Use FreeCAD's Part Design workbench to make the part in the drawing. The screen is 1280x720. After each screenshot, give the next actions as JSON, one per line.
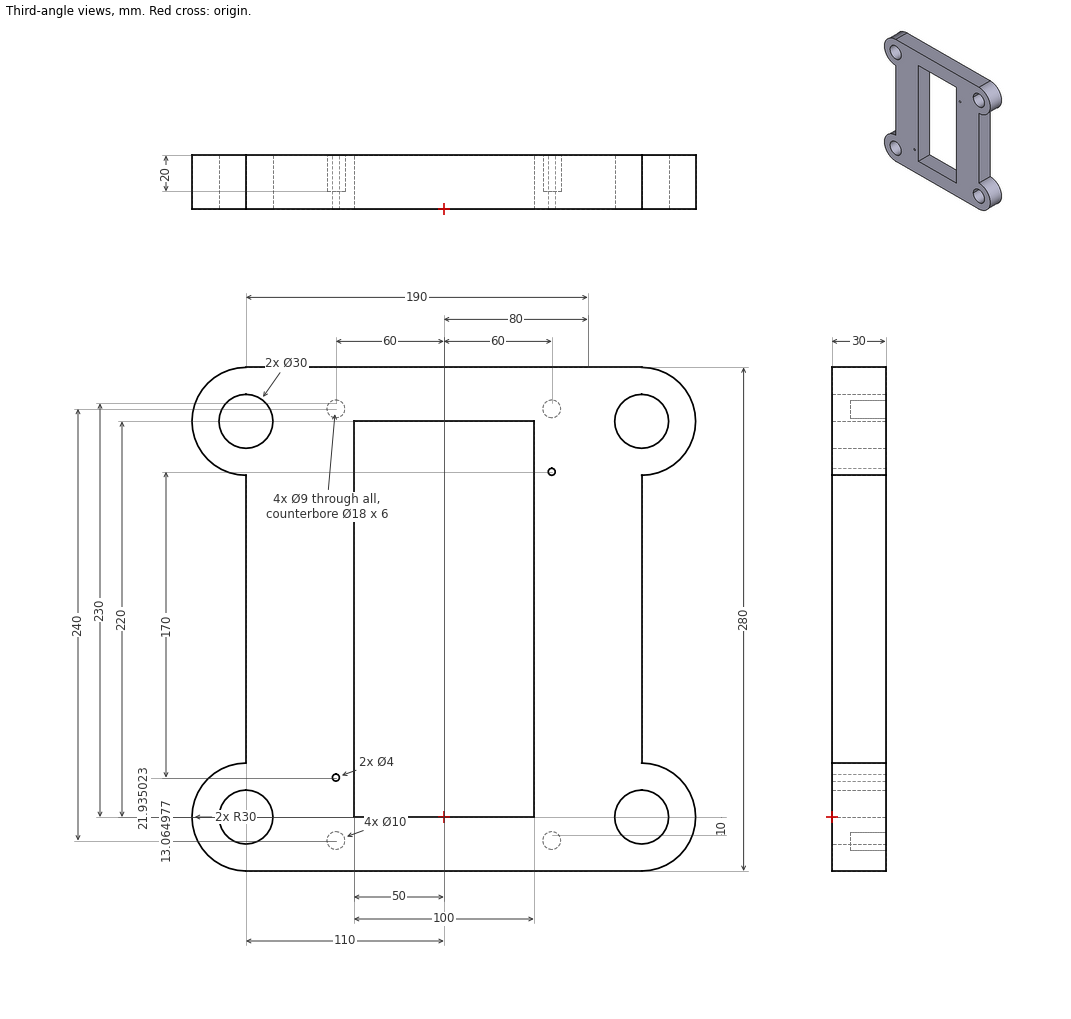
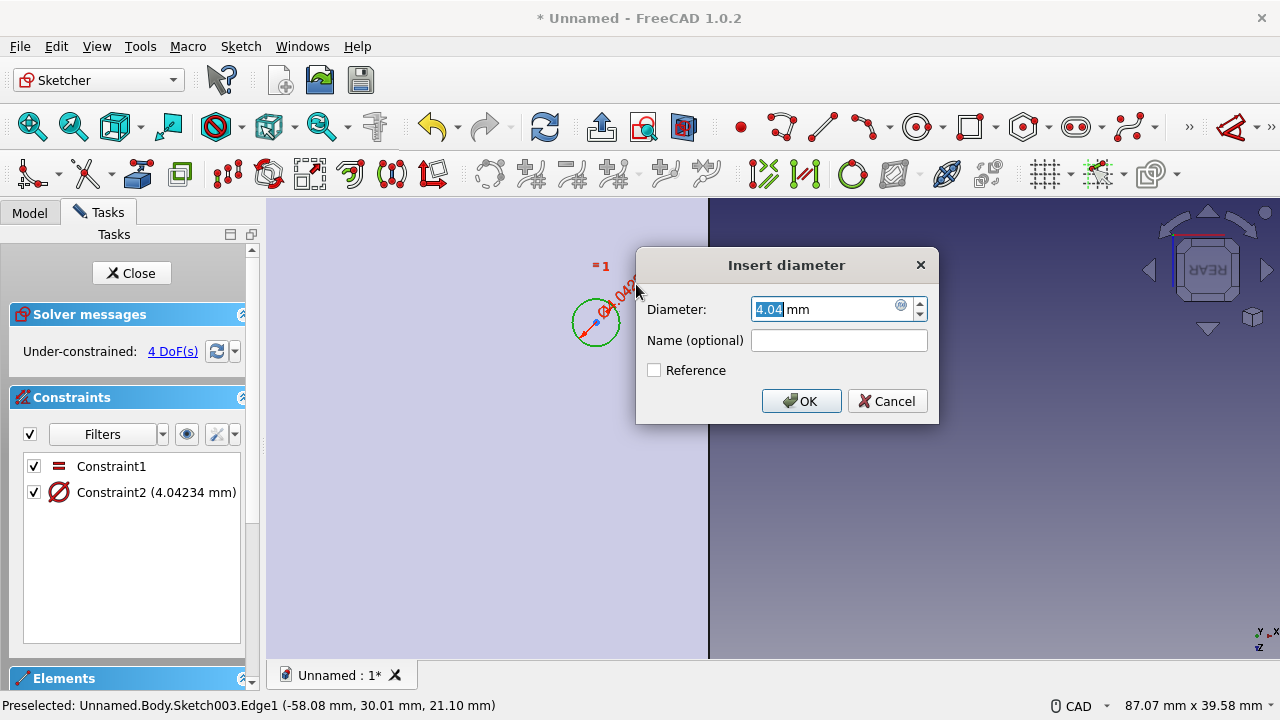
{"action": "type", "text": "4"}
{"action": "key", "text": "Return"}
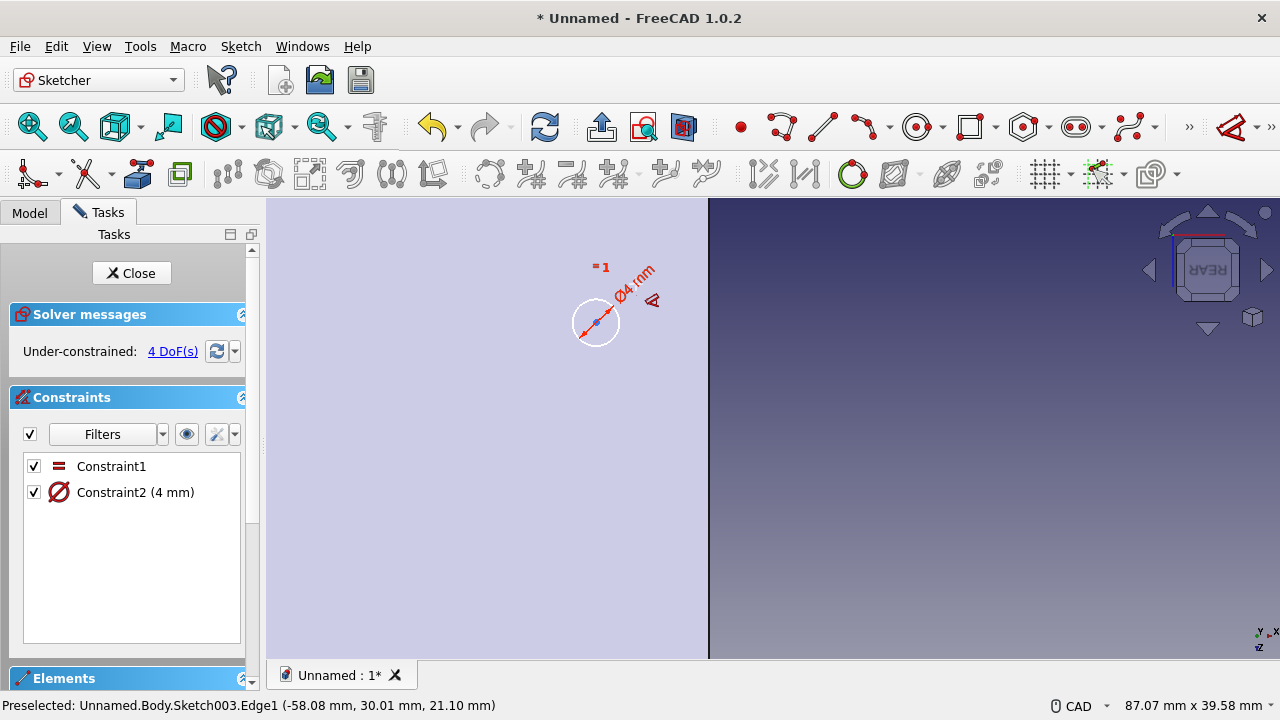
{"action": "scroll", "coordinate": [613, 309], "scroll_direction": "down", "scroll_amount": 10}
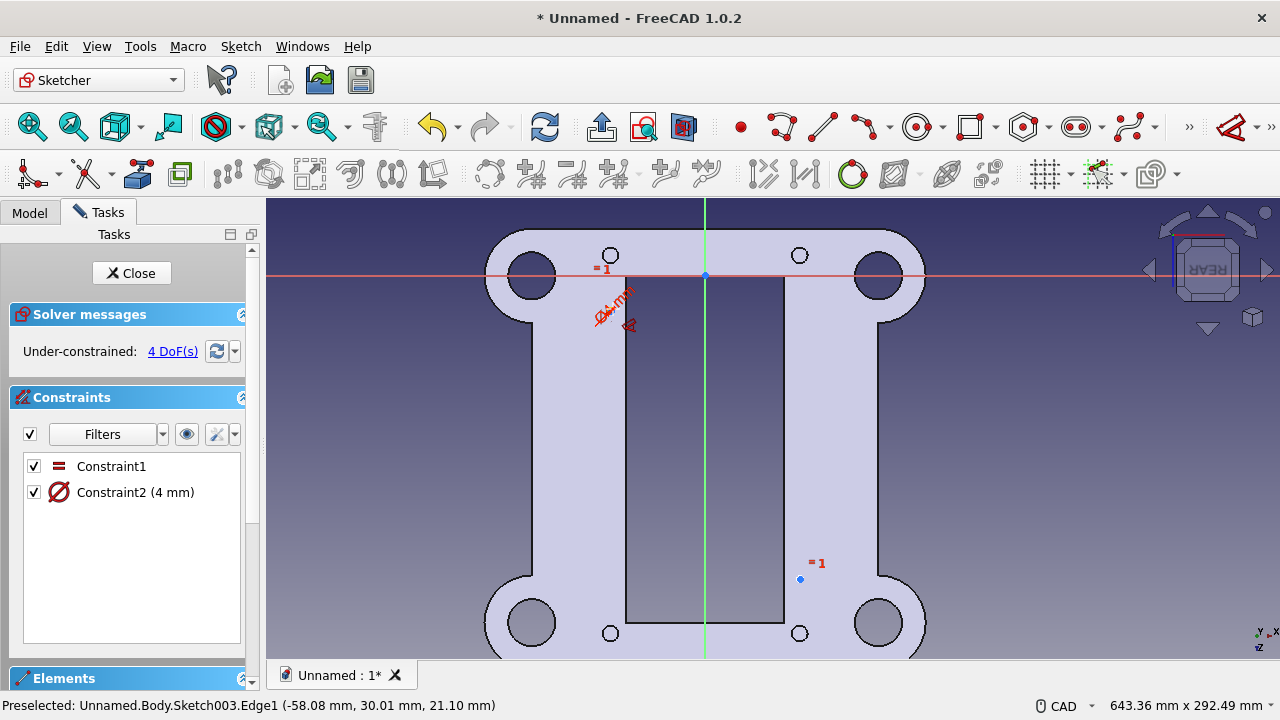
{"action": "left_click", "coordinate": [611, 311]}
{"action": "left_click", "coordinate": [658, 242]}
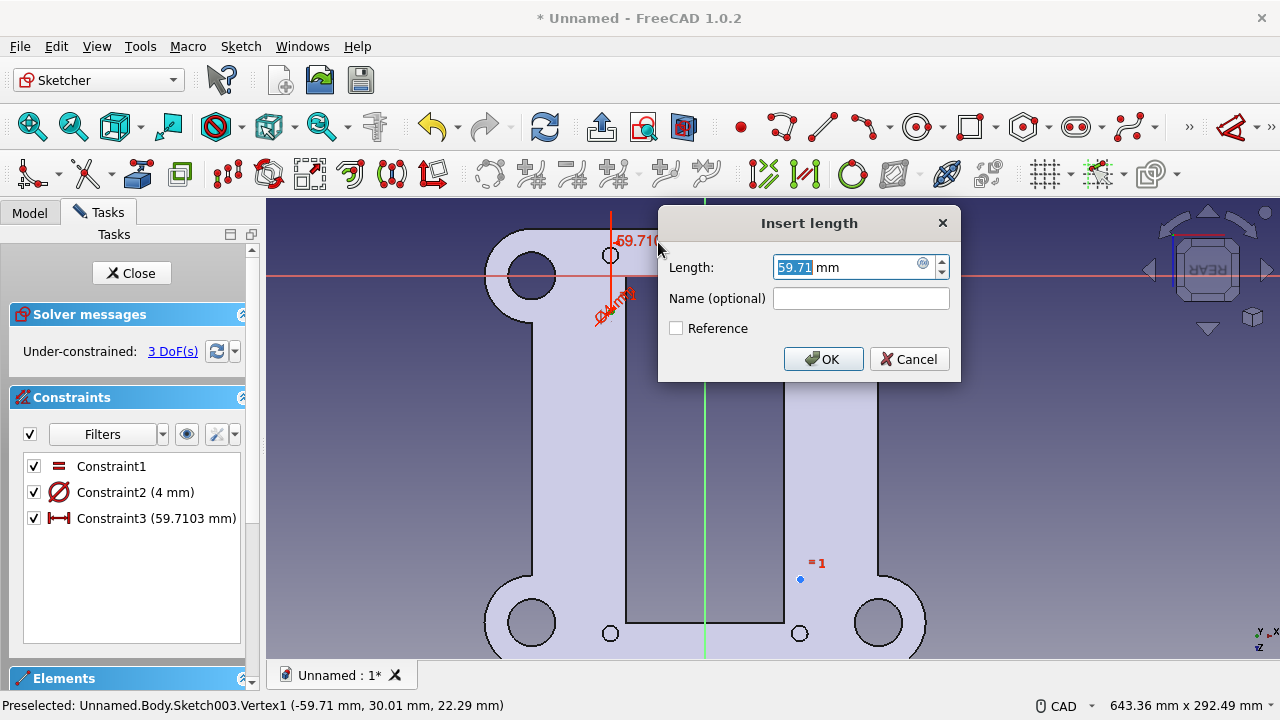
{"action": "type", "text": "60"}
{"action": "key", "text": "Return"}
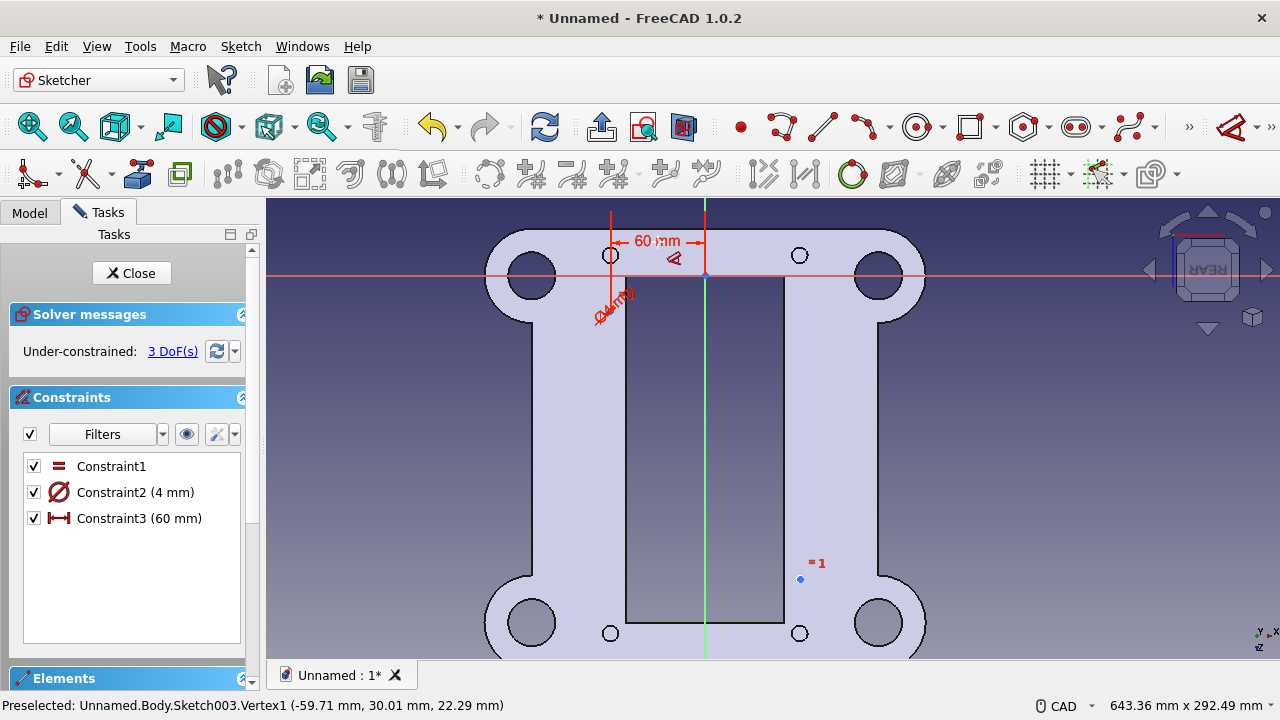
{"action": "left_click", "coordinate": [800, 579]}
{"action": "left_click", "coordinate": [753, 242]}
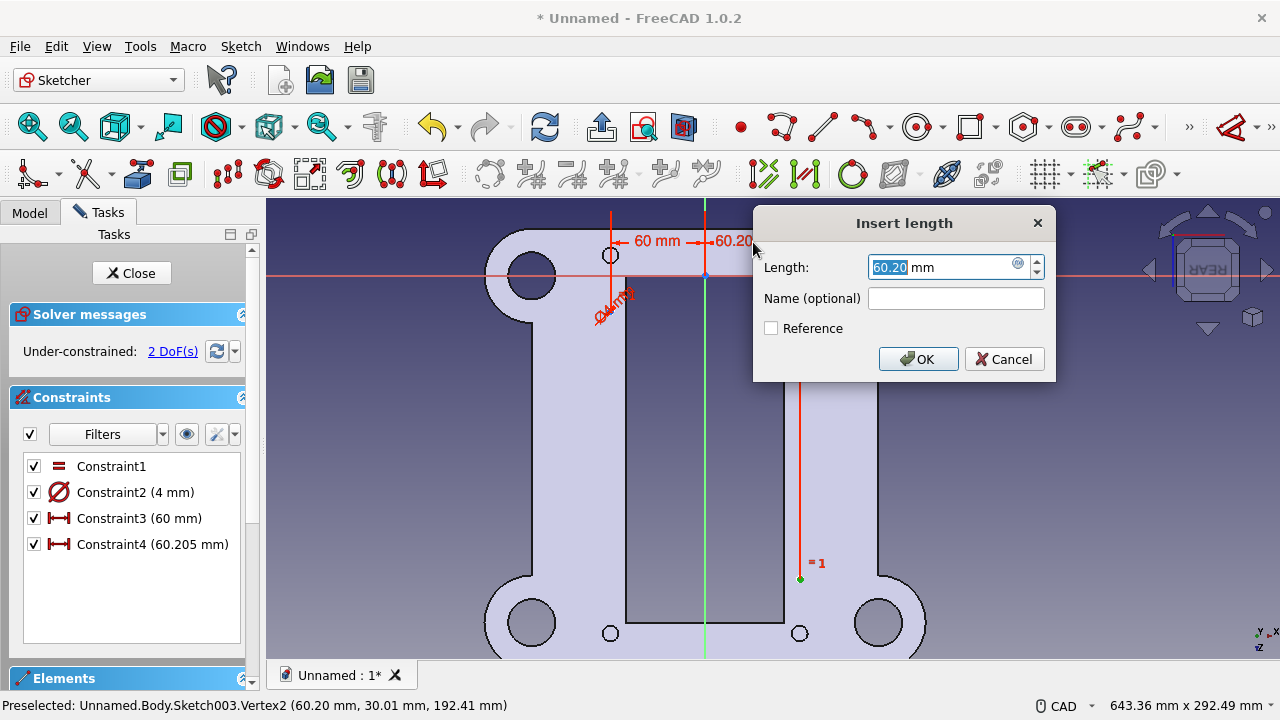
{"action": "type", "text": "60"}
{"action": "key", "text": "Return"}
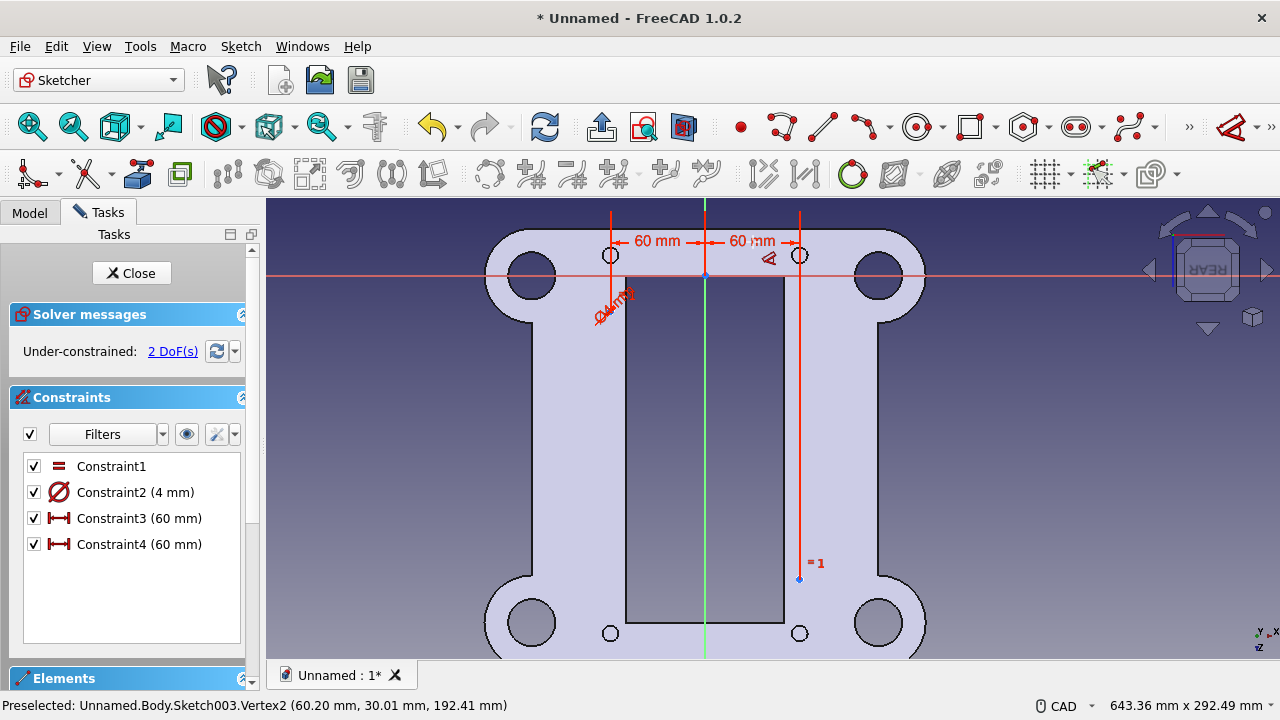
{"action": "left_click", "coordinate": [611, 311]}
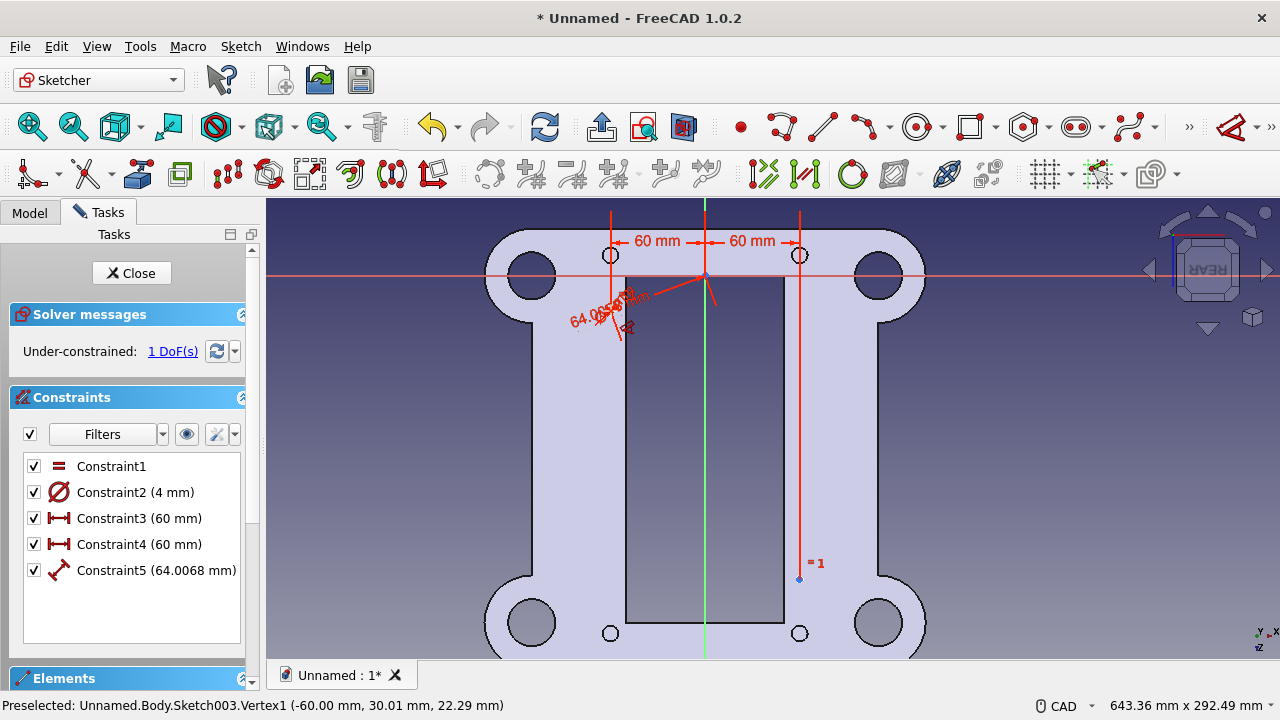
{"action": "left_click", "coordinate": [800, 579]}
{"action": "left_click", "coordinate": [834, 445]}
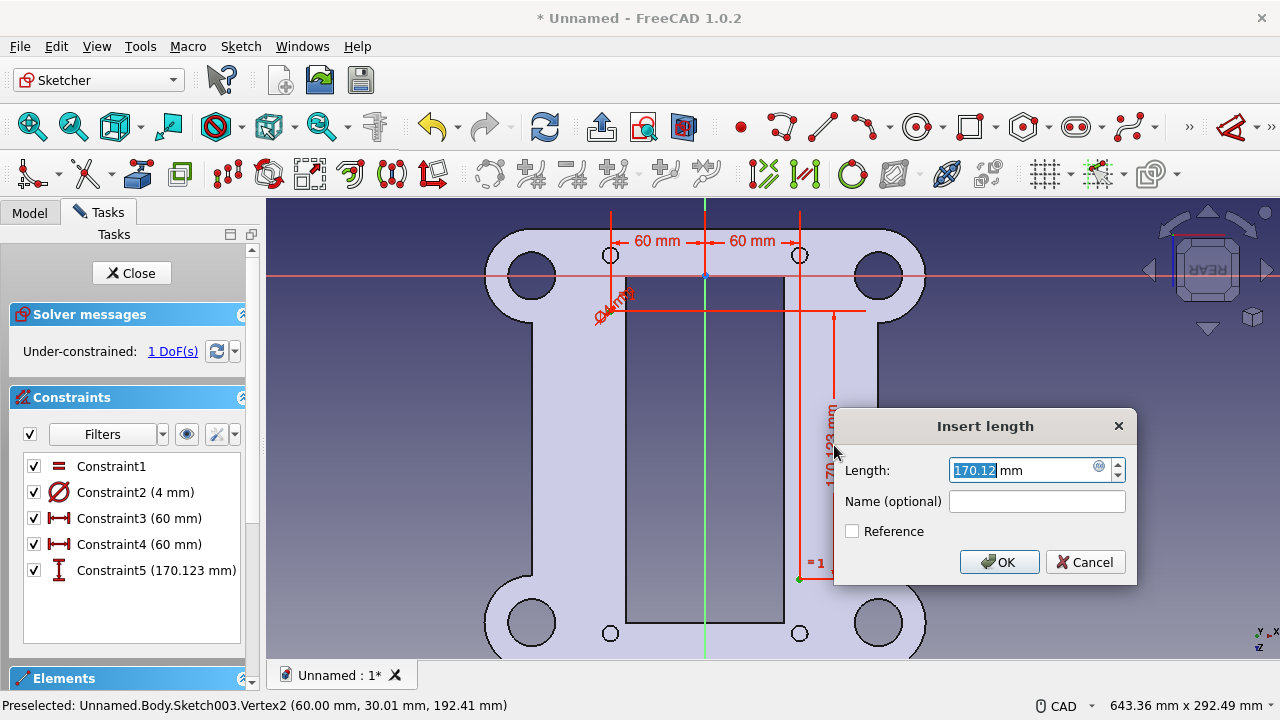
{"action": "type", "text": "170"}
{"action": "key", "text": "Return"}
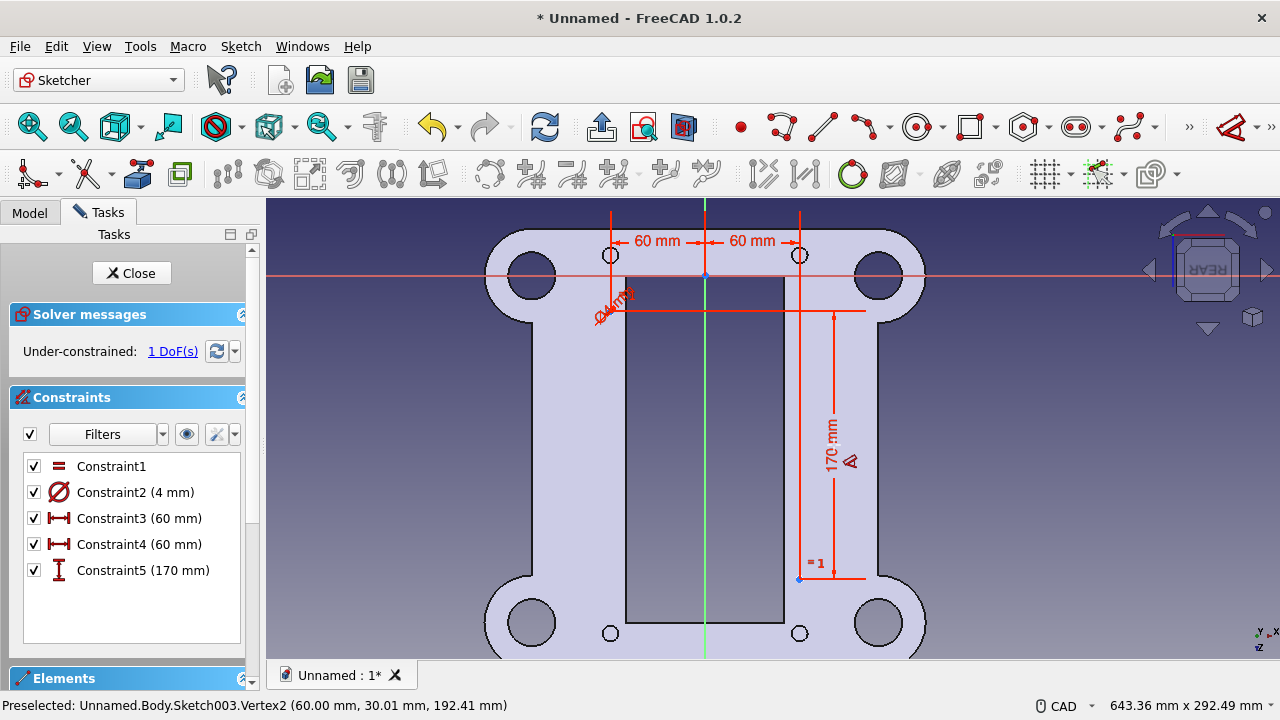
{"action": "left_click", "coordinate": [611, 311]}
{"action": "left_click", "coordinate": [739, 294]}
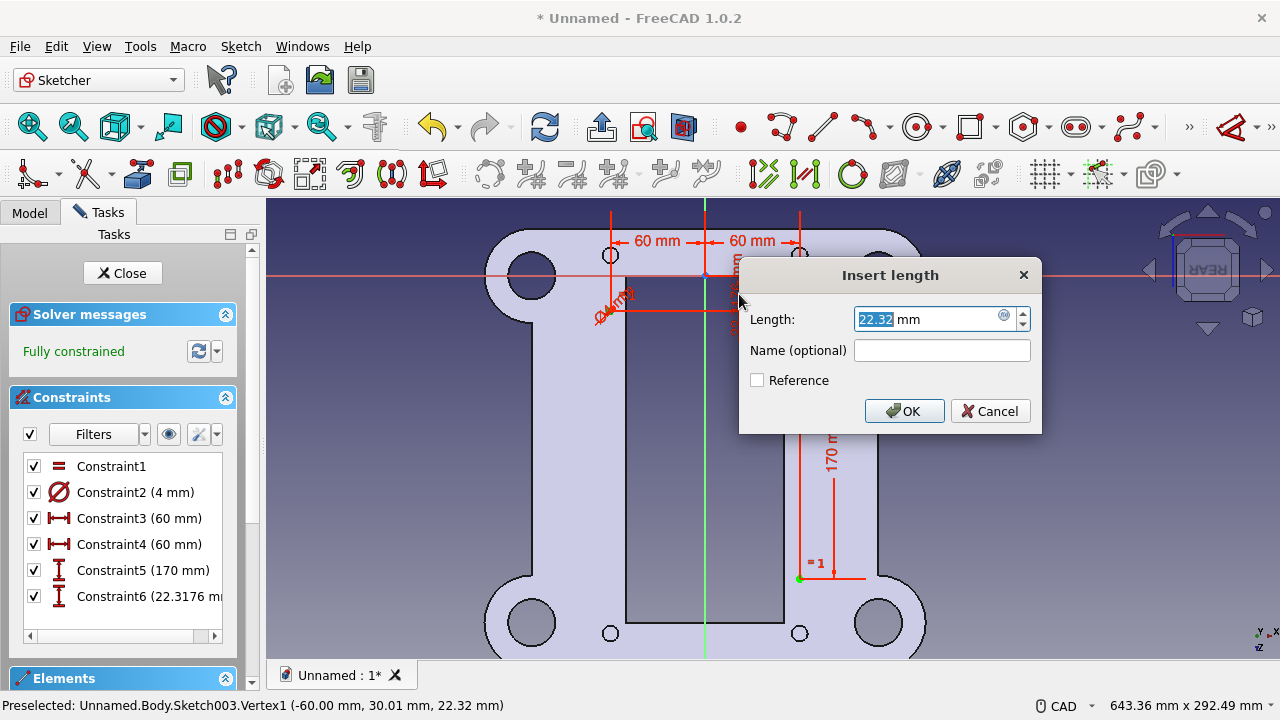
{"action": "type", "text": "21.935023"}
{"action": "key", "text": "Return"}
{"action": "key", "text": "Escape"}